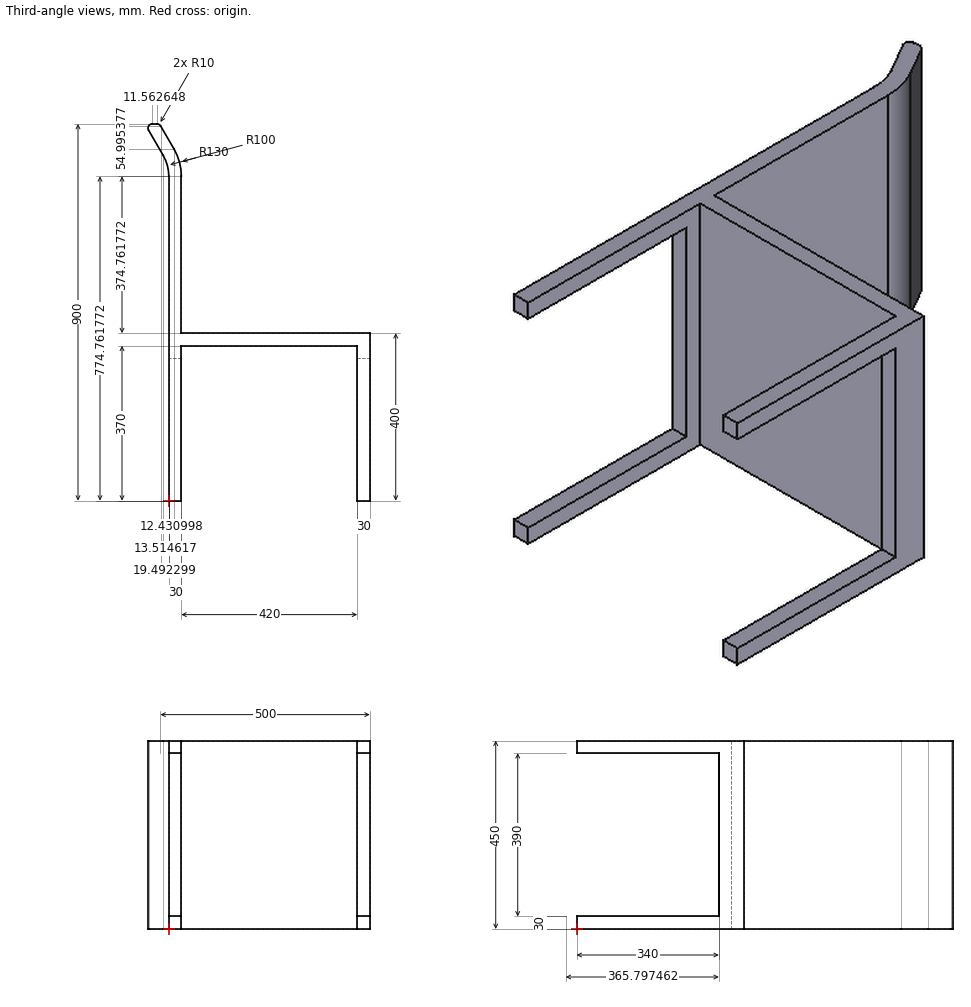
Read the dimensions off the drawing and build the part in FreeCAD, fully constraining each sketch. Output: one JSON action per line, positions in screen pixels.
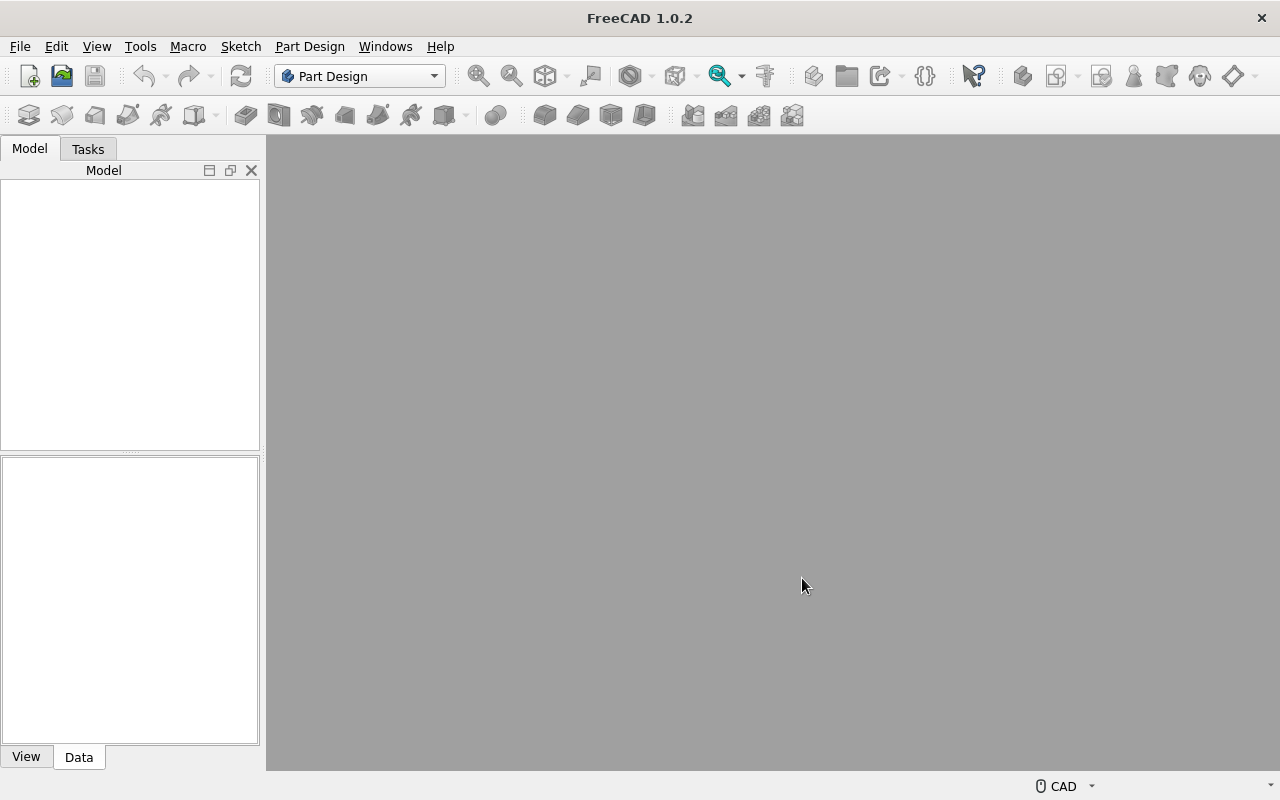
{"action": "left_click", "coordinate": [29, 76]}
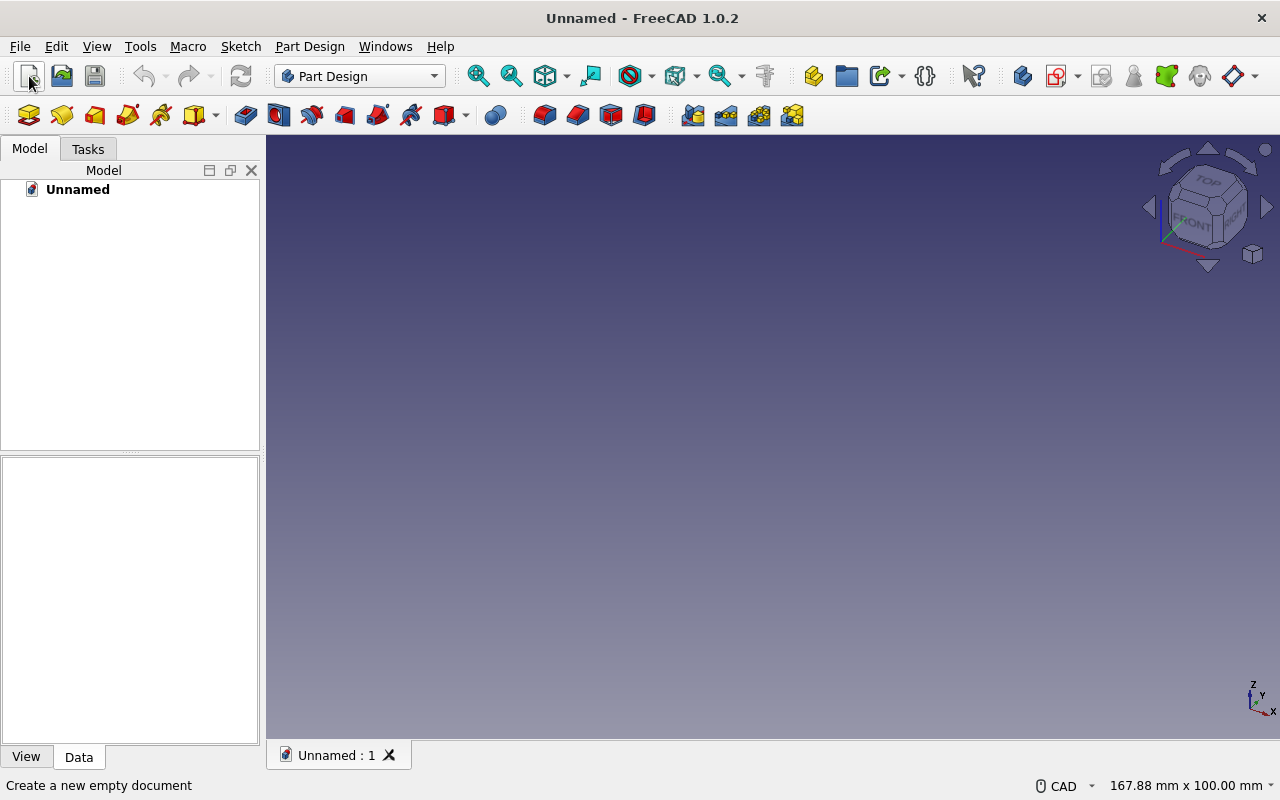
{"action": "left_click", "coordinate": [1056, 76]}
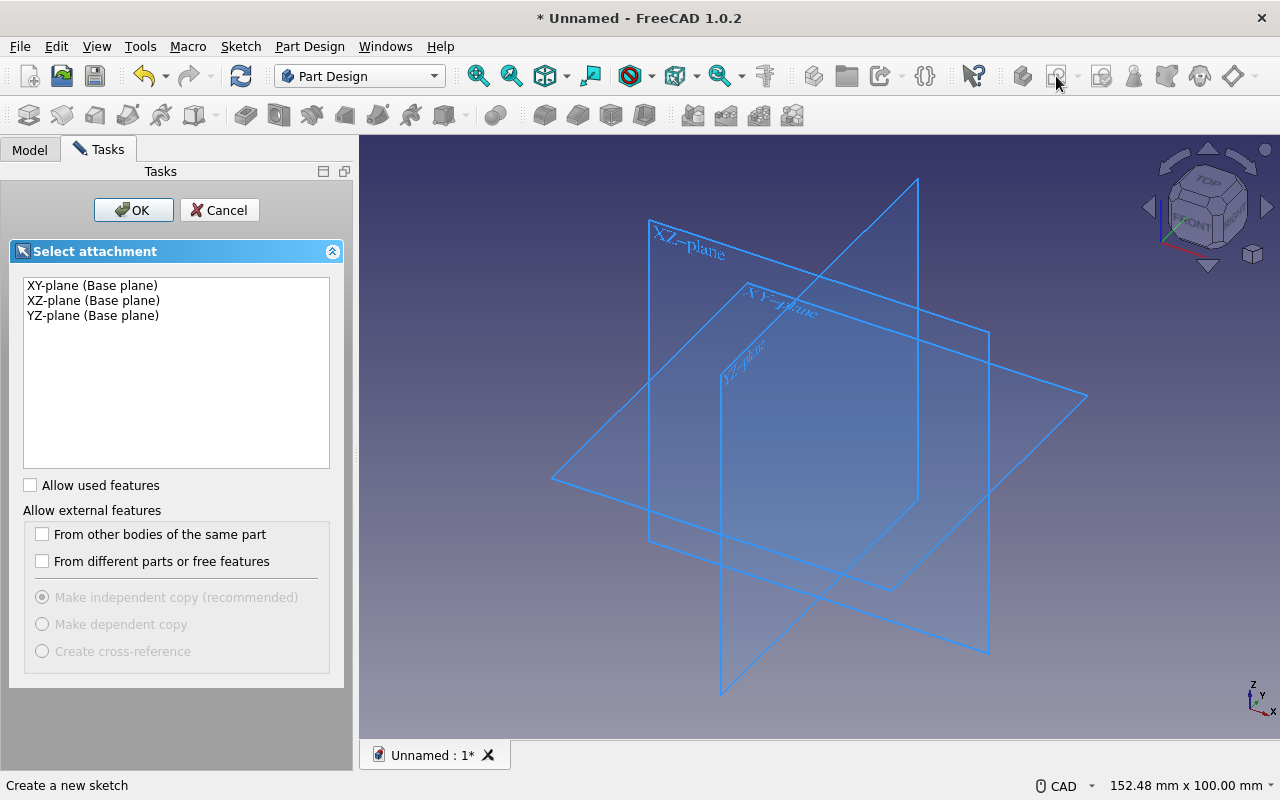
{"action": "left_click", "coordinate": [84, 286]}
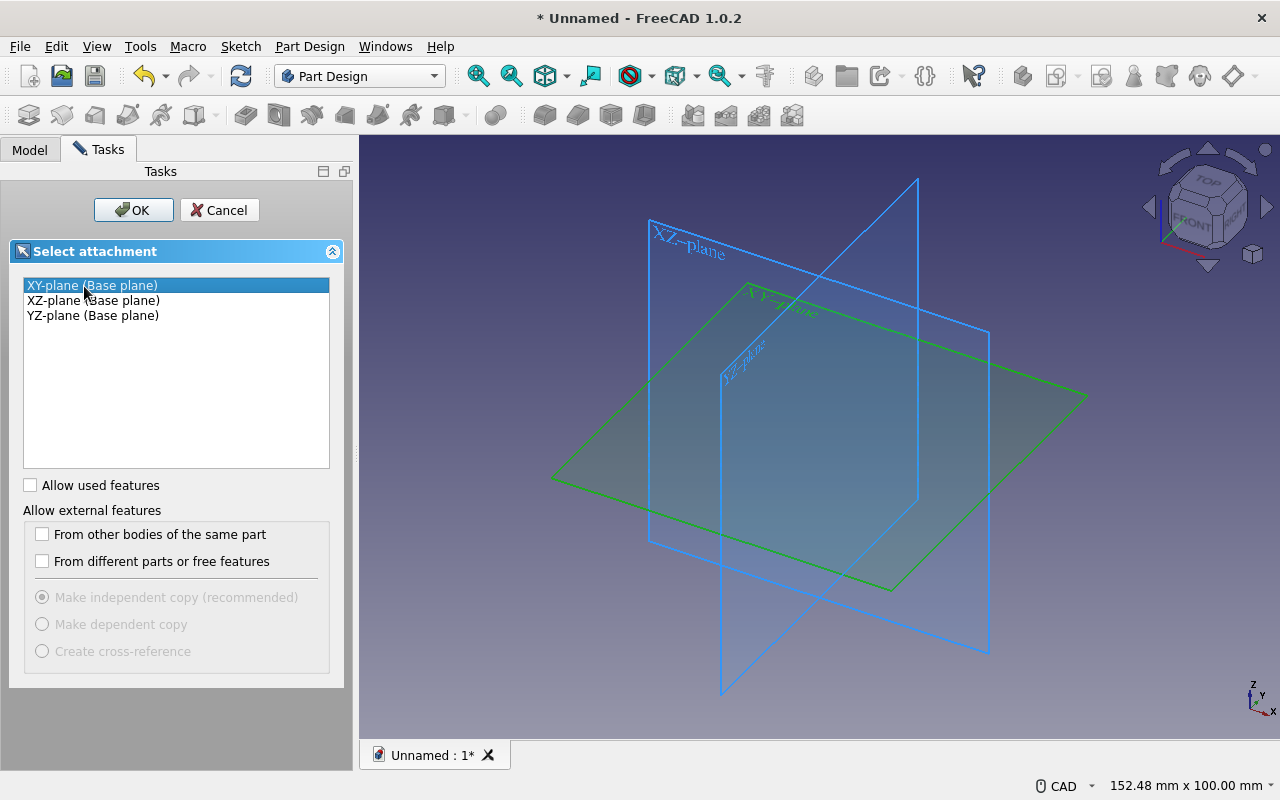
{"action": "left_click", "coordinate": [134, 210]}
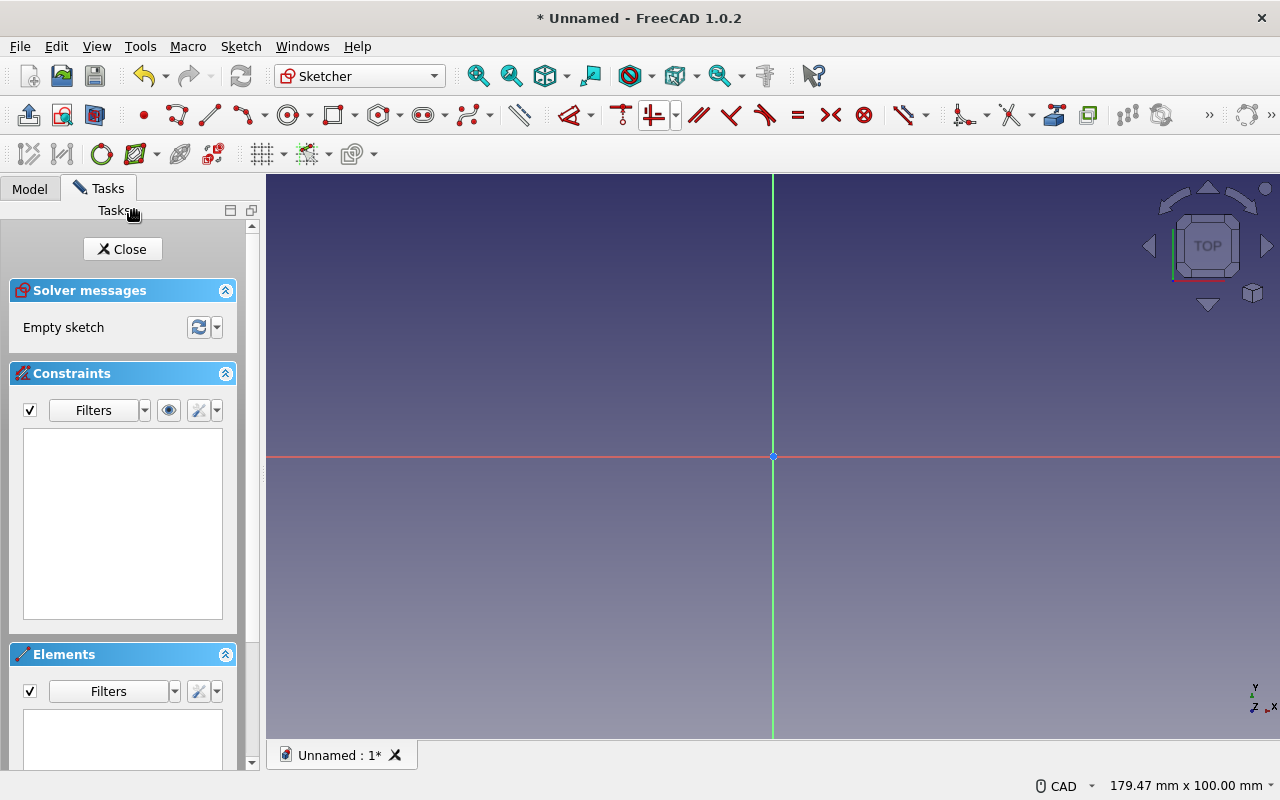
{"action": "scroll", "coordinate": [601, 660], "scroll_direction": "down", "scroll_amount": 13}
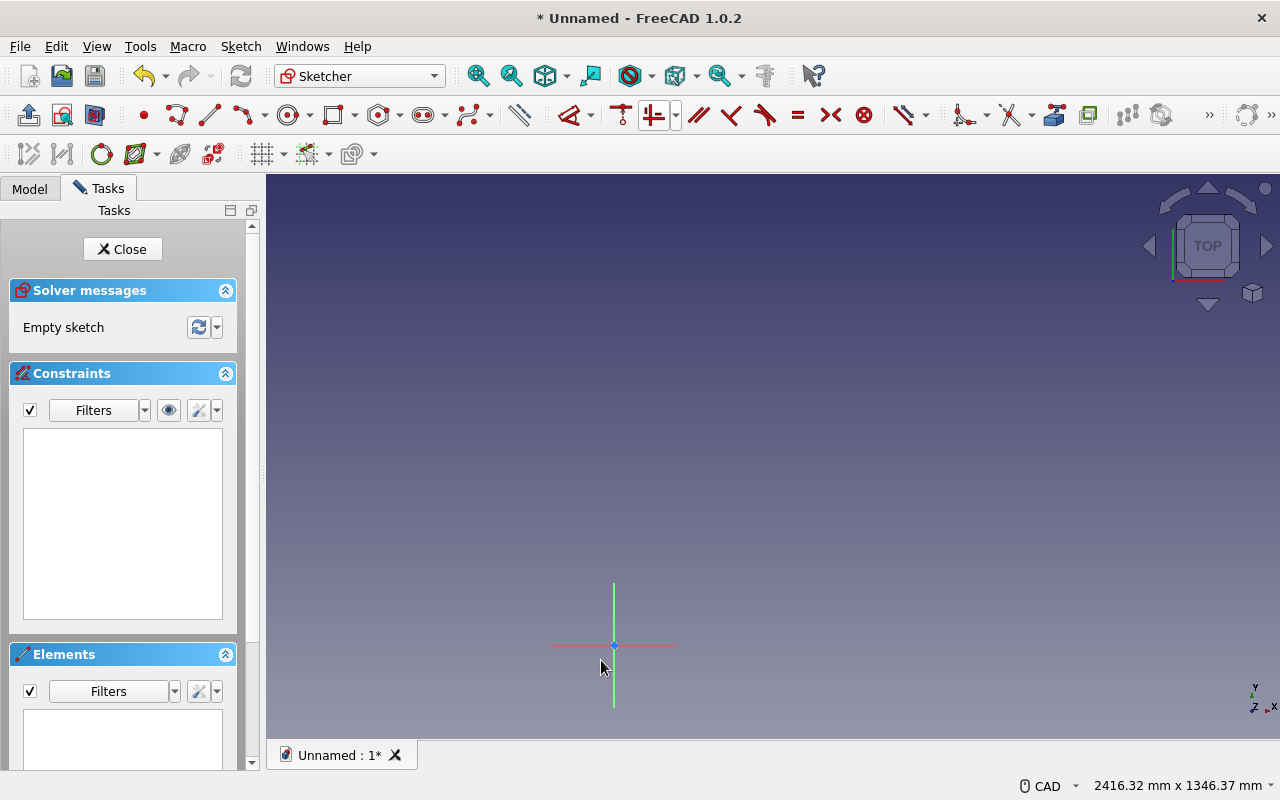
{"action": "left_click", "coordinate": [177, 116]}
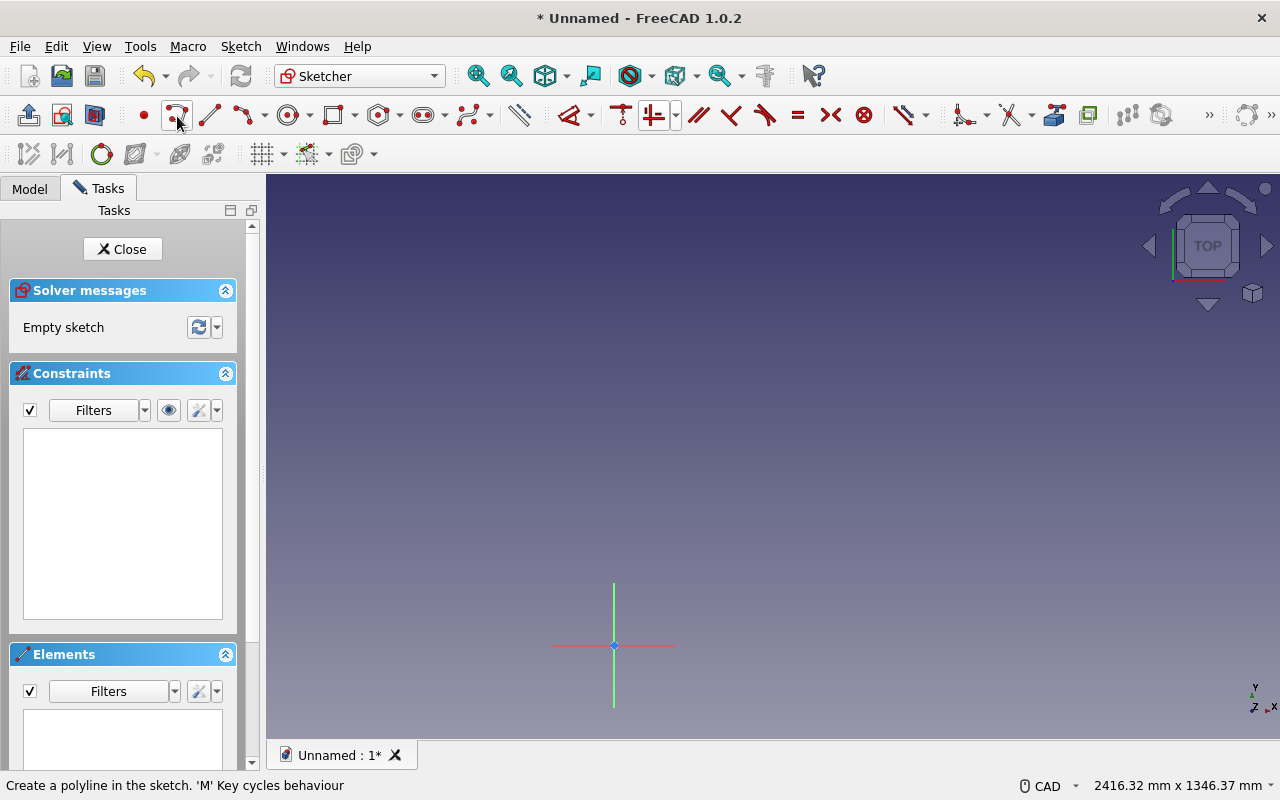
{"action": "left_click", "coordinate": [614, 321]}
{"action": "left_click", "coordinate": [614, 646]}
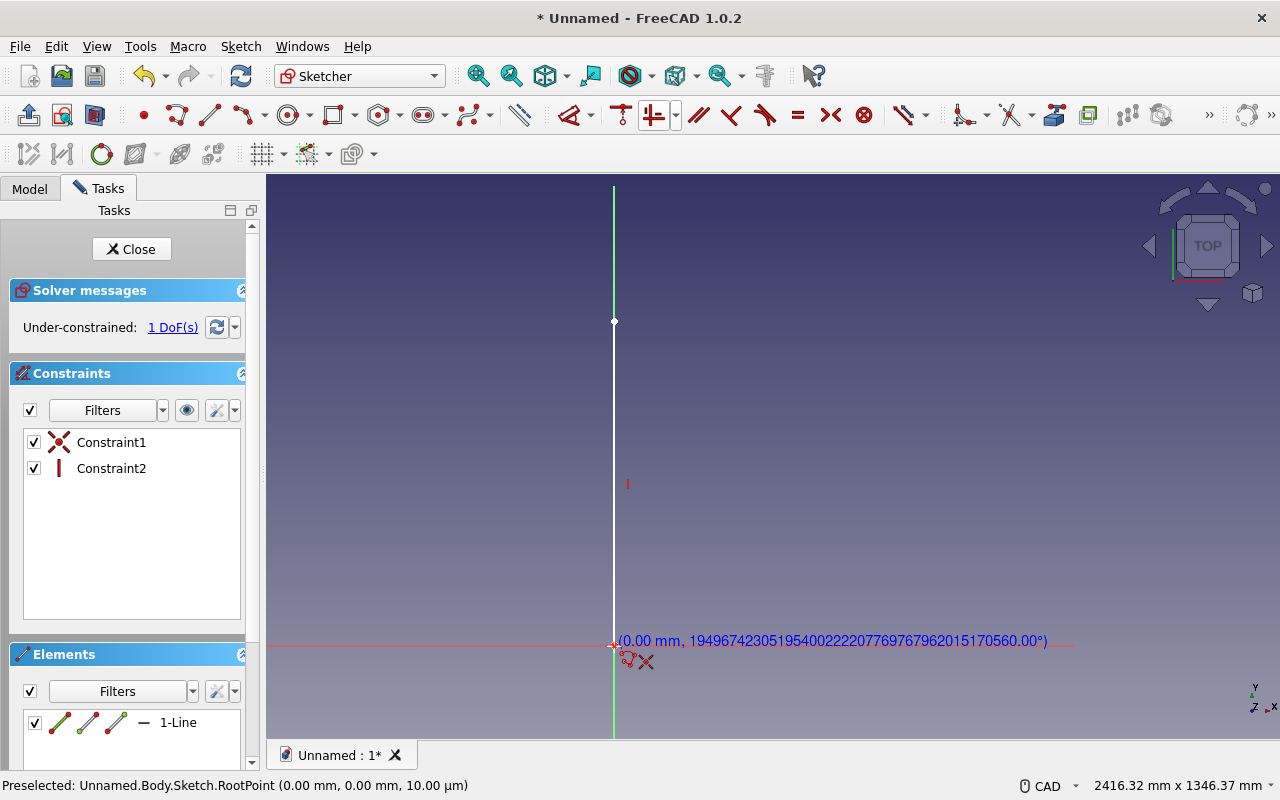
{"action": "scroll", "coordinate": [627, 646], "scroll_direction": "up", "scroll_amount": 2}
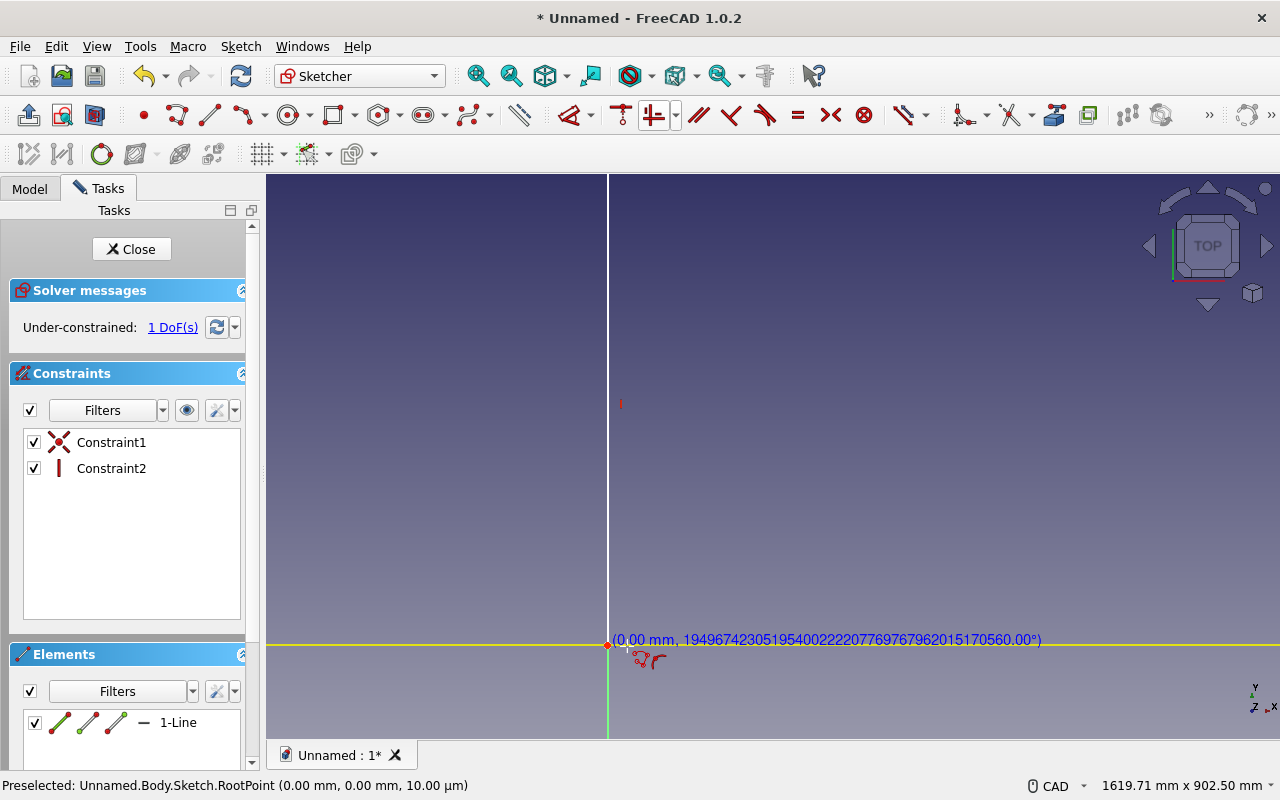
{"action": "left_click", "coordinate": [626, 636]}
{"action": "left_click", "coordinate": [626, 413]}
{"action": "left_click", "coordinate": [889, 413]}
{"action": "left_click", "coordinate": [889, 645]}
{"action": "left_click", "coordinate": [908, 636]}
{"action": "left_click", "coordinate": [908, 395]}
{"action": "left_click", "coordinate": [626, 395]}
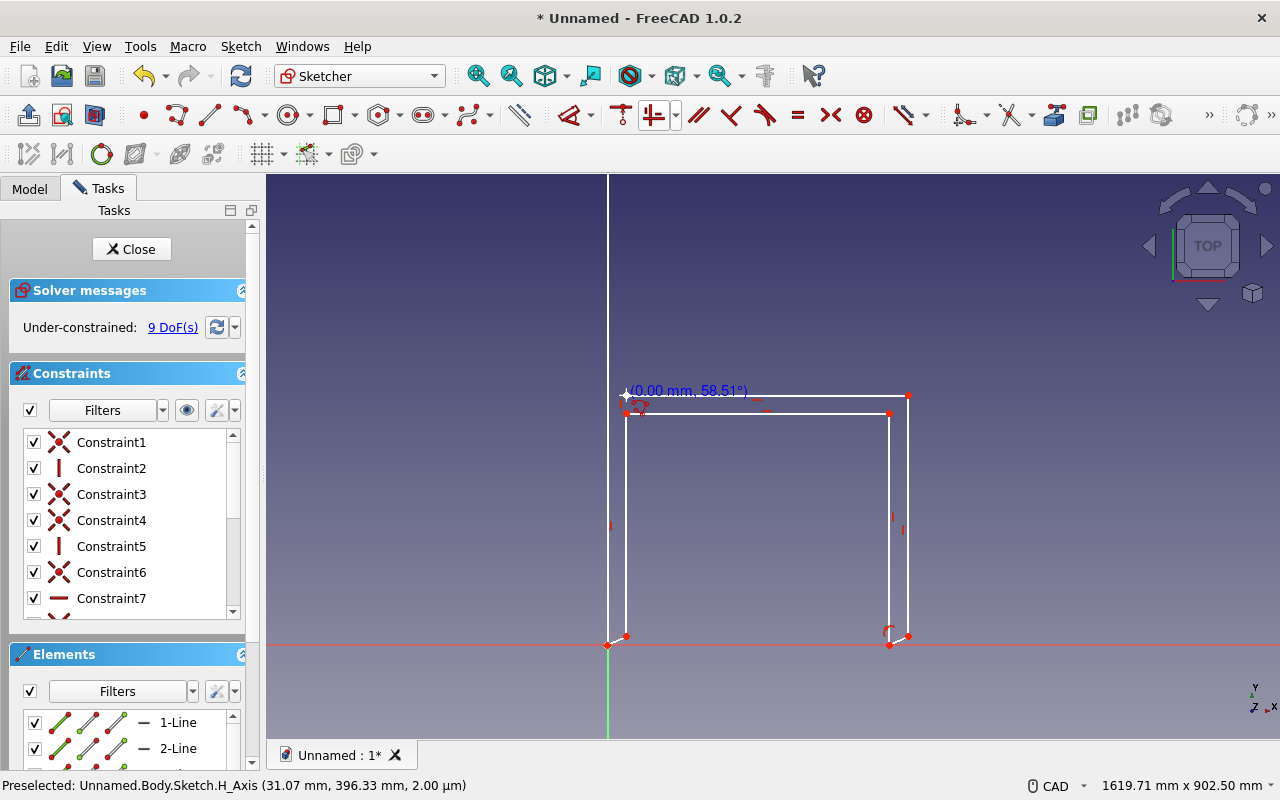
{"action": "scroll", "coordinate": [627, 646], "scroll_direction": "down", "scroll_amount": 2}